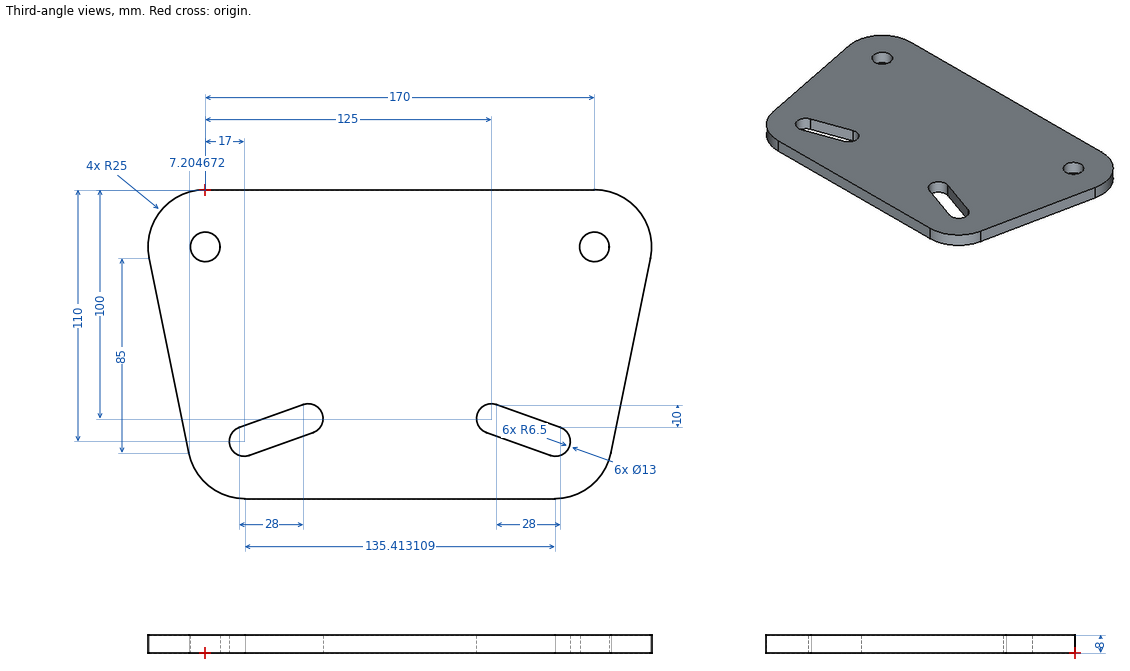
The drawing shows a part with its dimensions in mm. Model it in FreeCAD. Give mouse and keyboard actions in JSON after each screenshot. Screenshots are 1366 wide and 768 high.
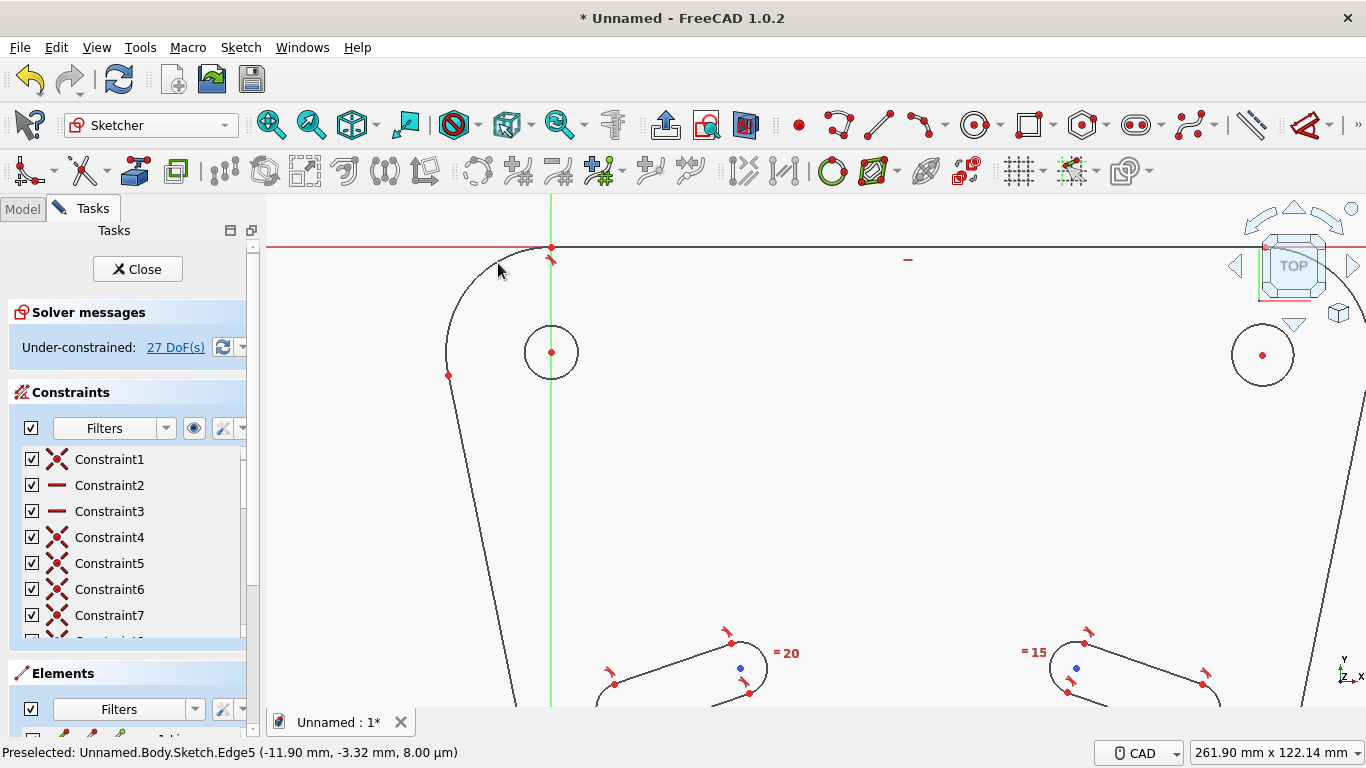
{"action": "left_click", "coordinate": [1051, 247]}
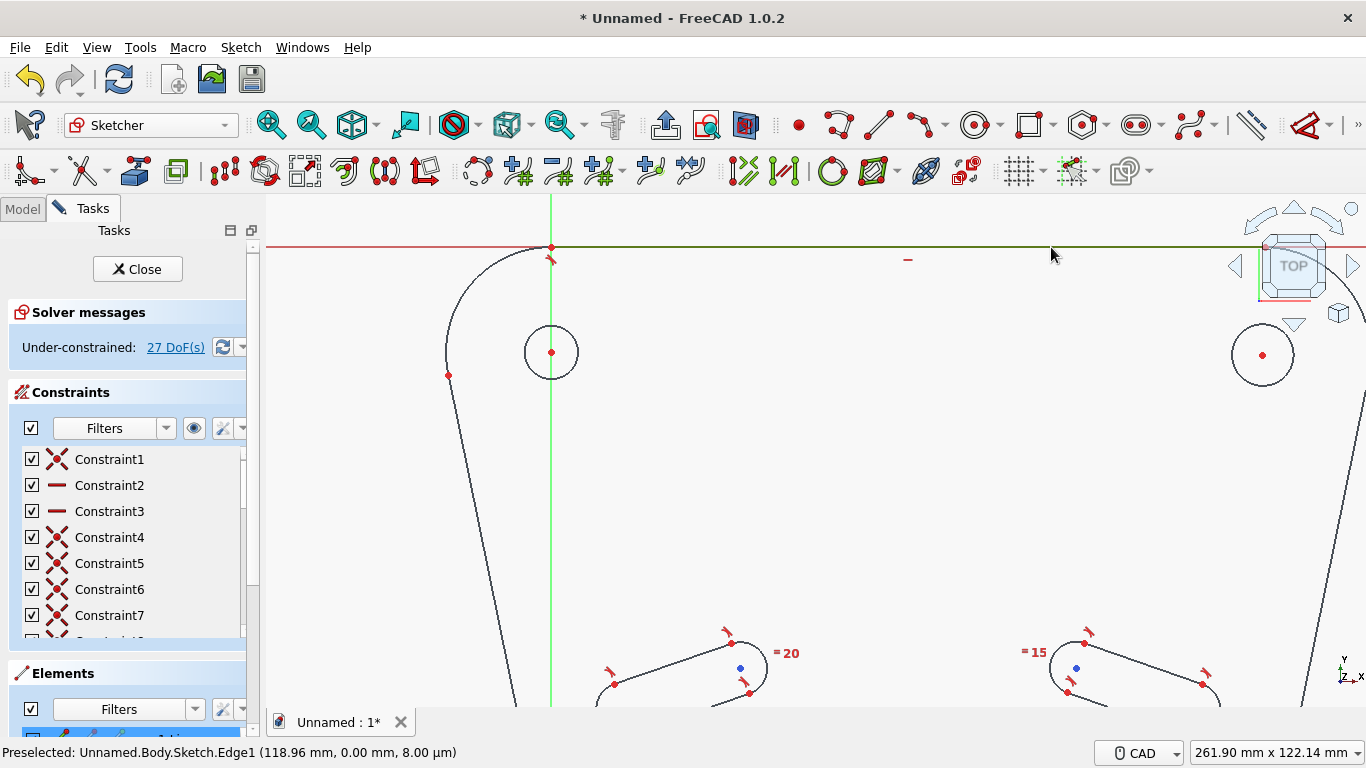
{"action": "scroll", "coordinate": [552, 353], "scroll_direction": "down", "scroll_amount": 3}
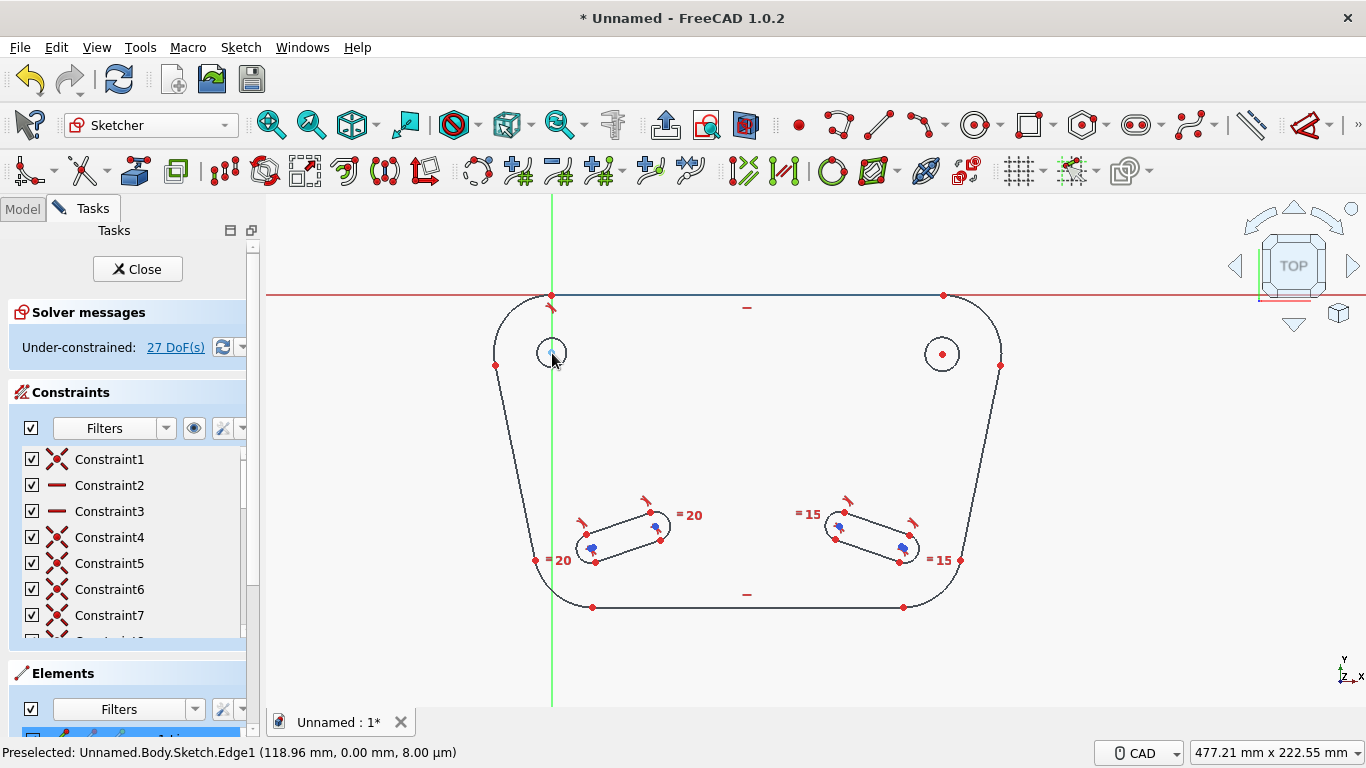
{"action": "left_click", "coordinate": [998, 335]}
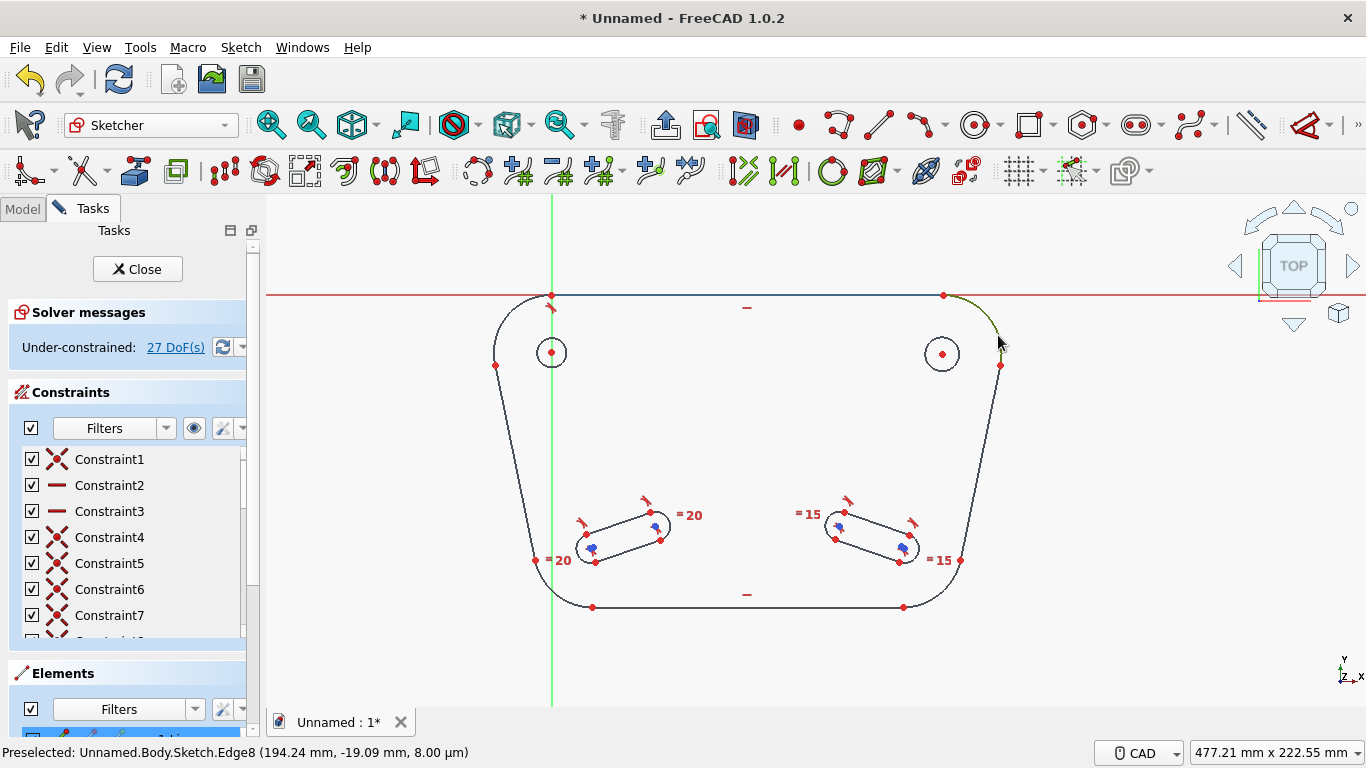
{"action": "key", "text": "t"}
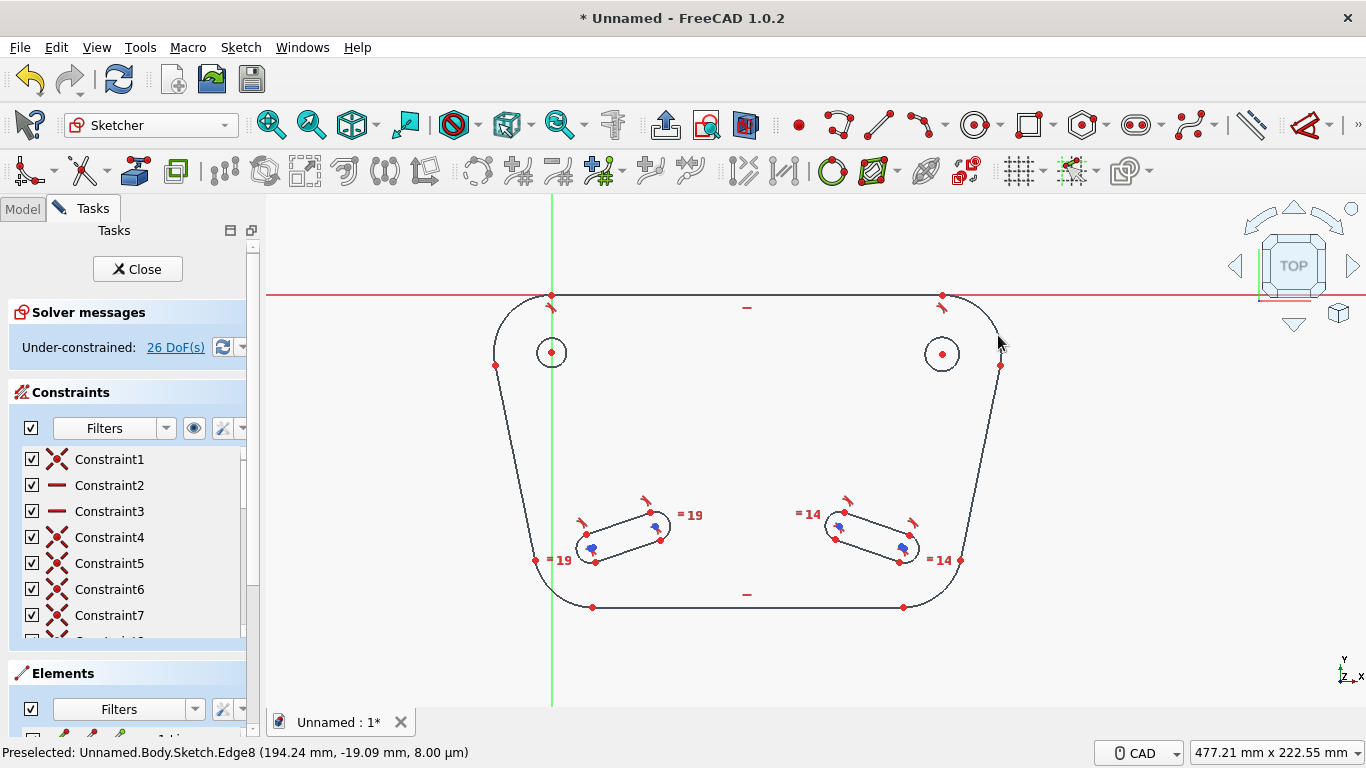
{"action": "left_click", "coordinate": [507, 424]}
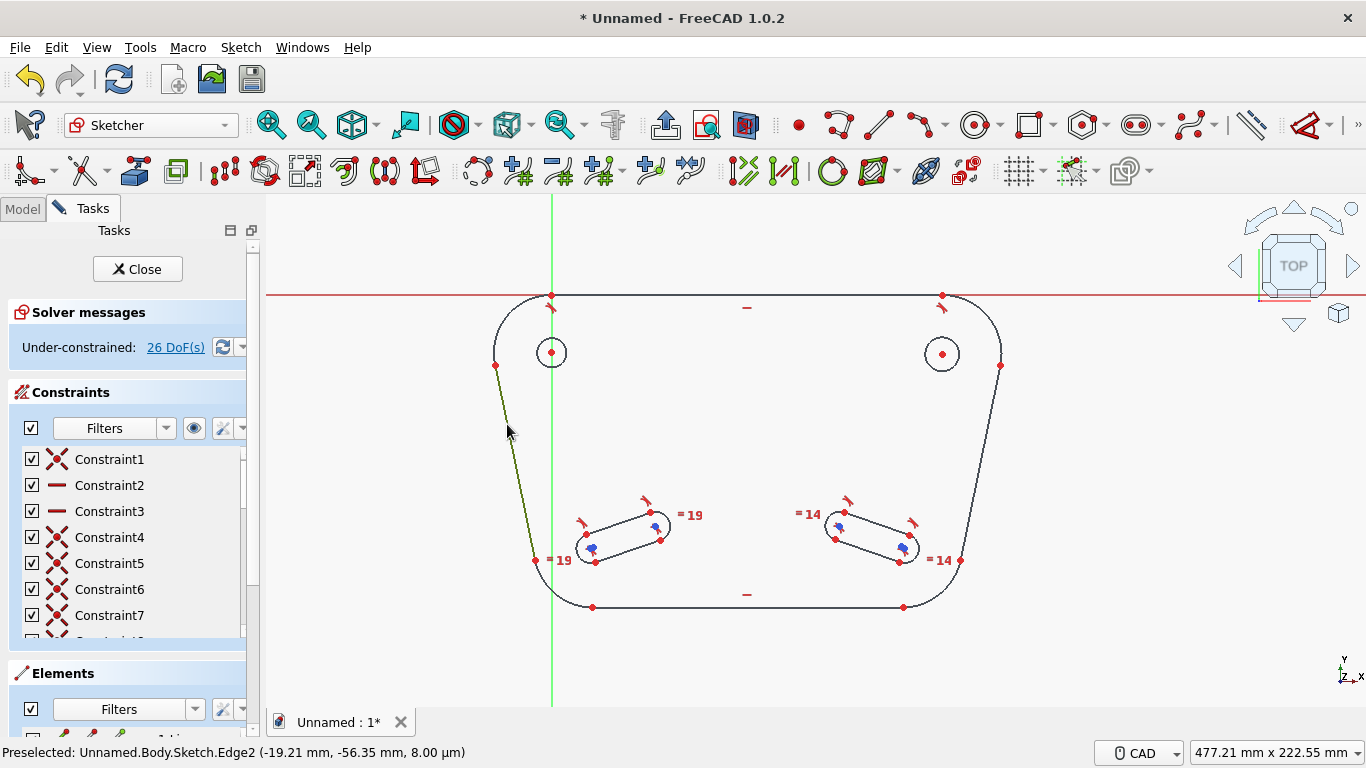
{"action": "left_click", "coordinate": [497, 335]}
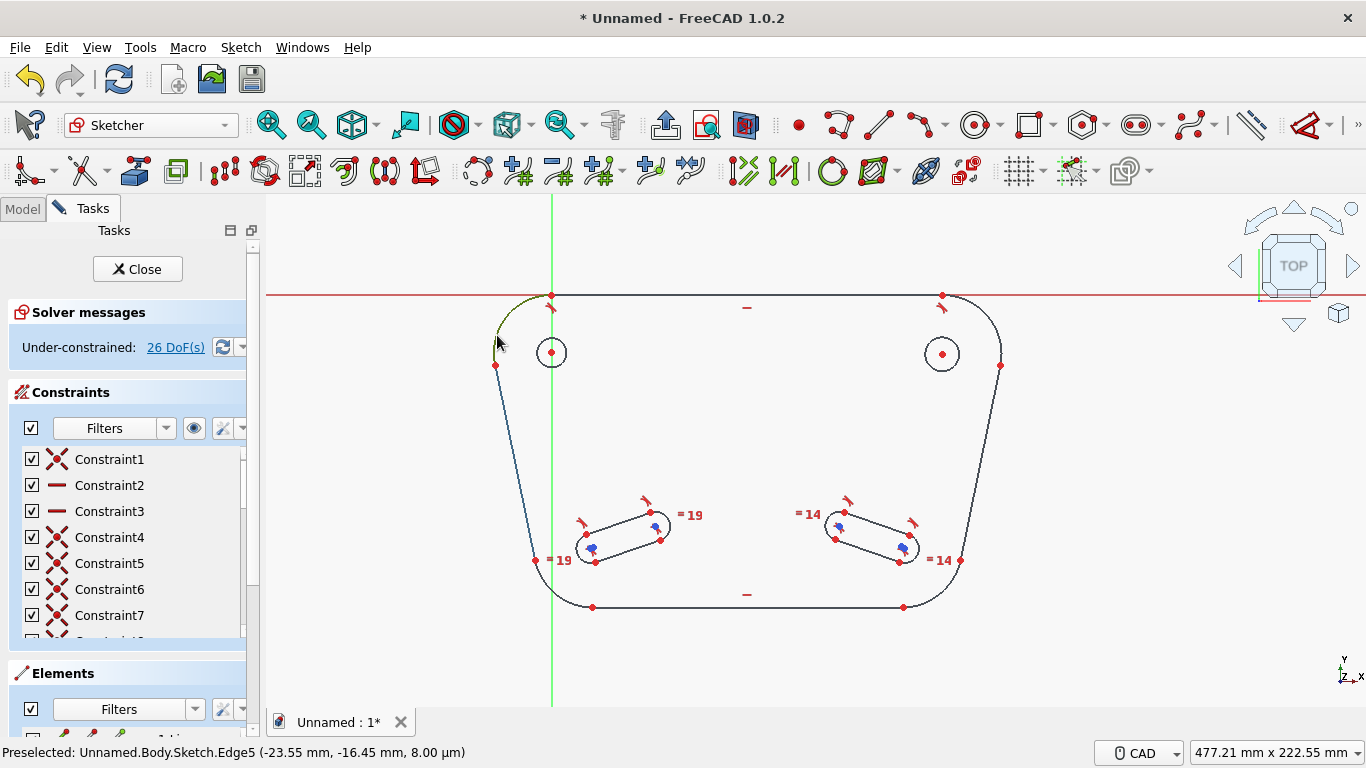
{"action": "key", "text": "t"}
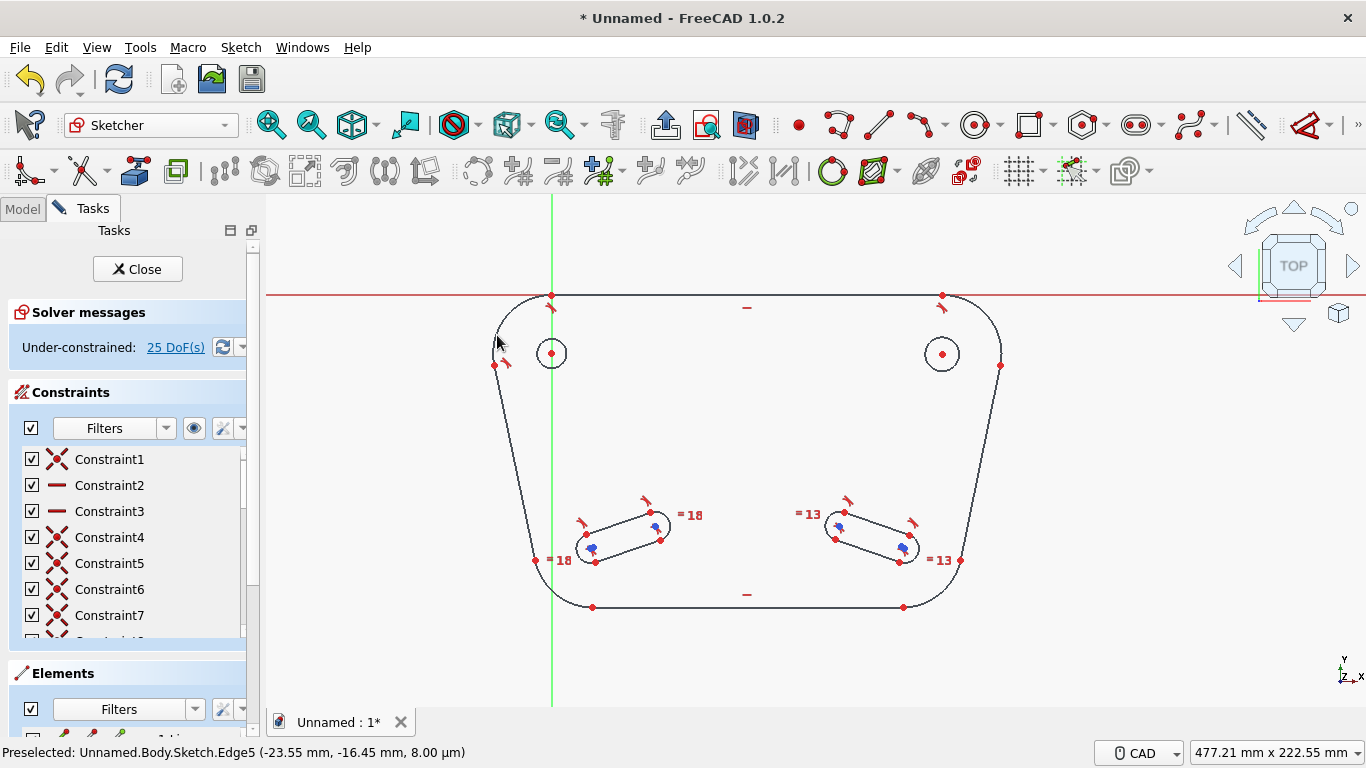
{"action": "left_click", "coordinate": [507, 424]}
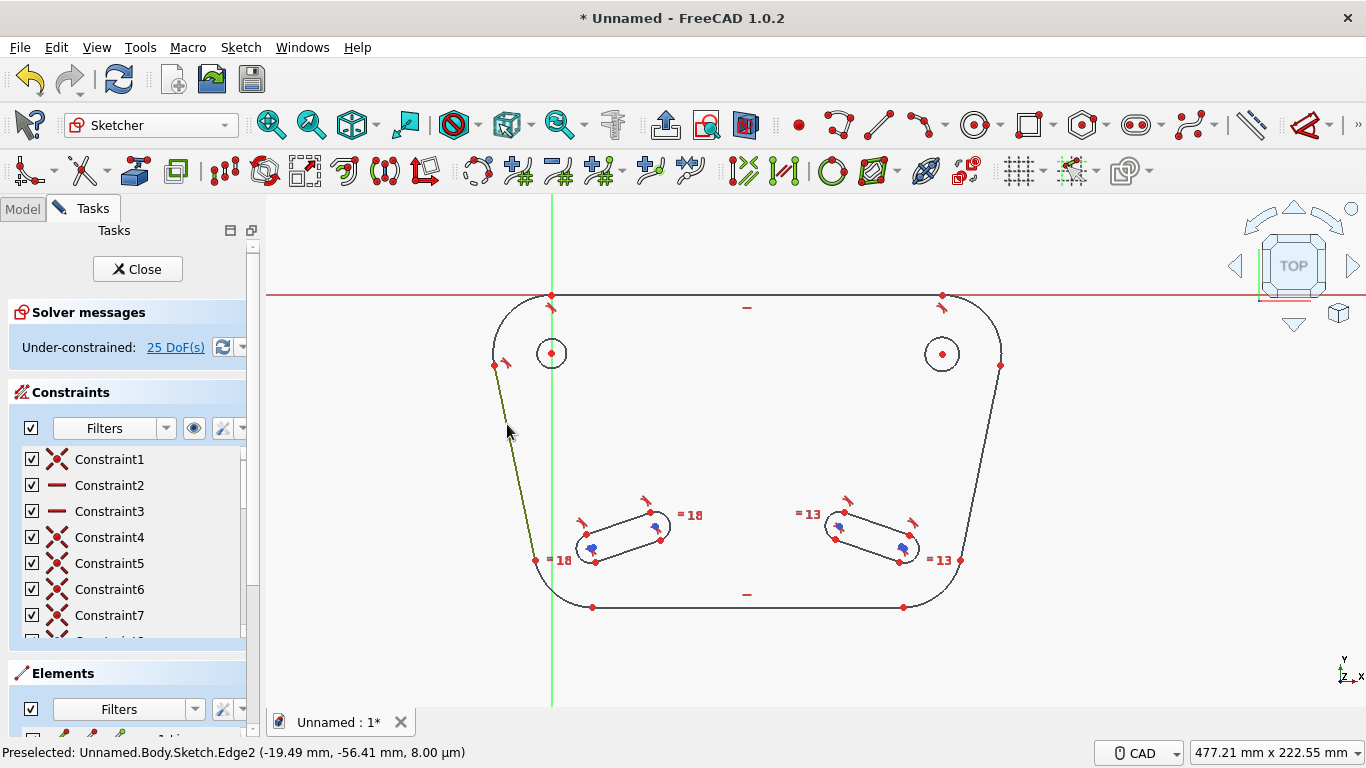
{"action": "left_click", "coordinate": [569, 602]}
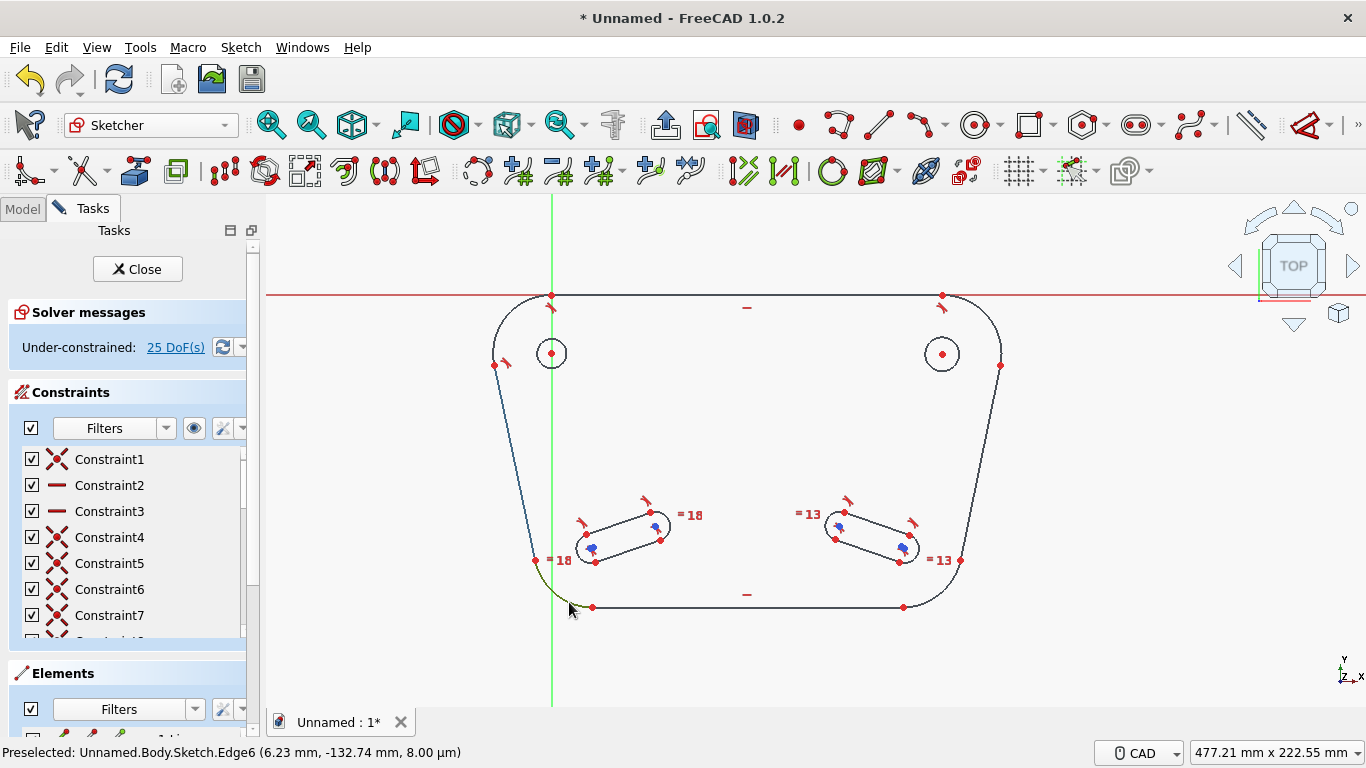
{"action": "key", "text": "t"}